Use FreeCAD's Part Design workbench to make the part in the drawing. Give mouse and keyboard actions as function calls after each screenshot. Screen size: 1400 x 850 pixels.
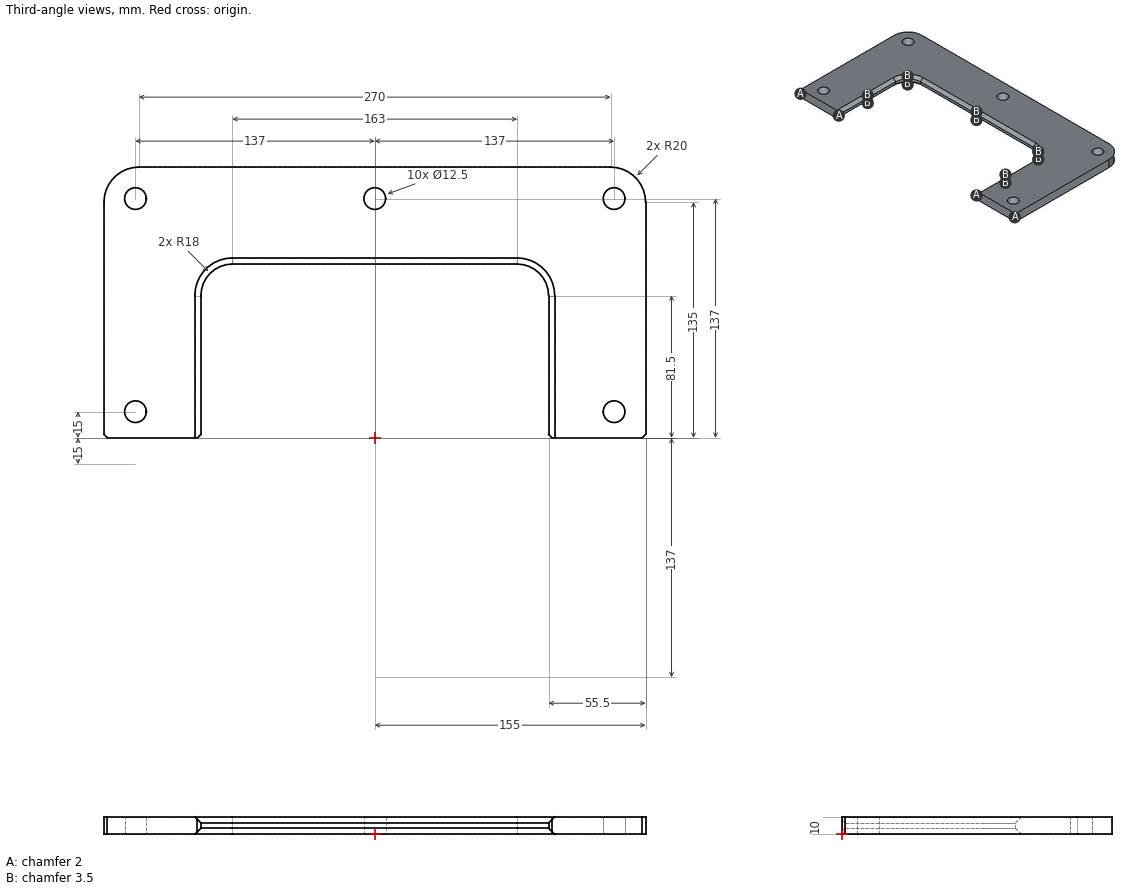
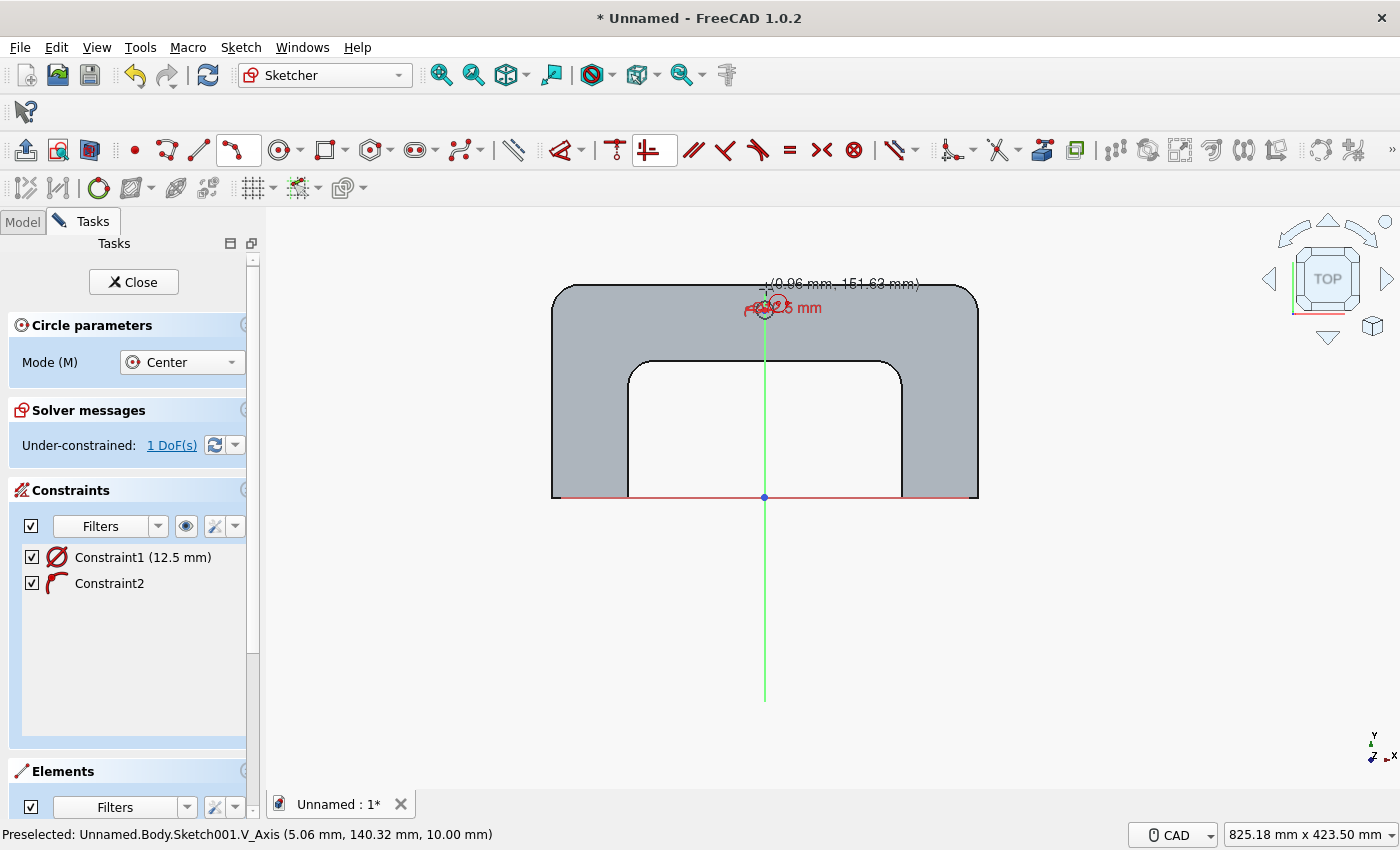
scroll(765, 686, up, 5)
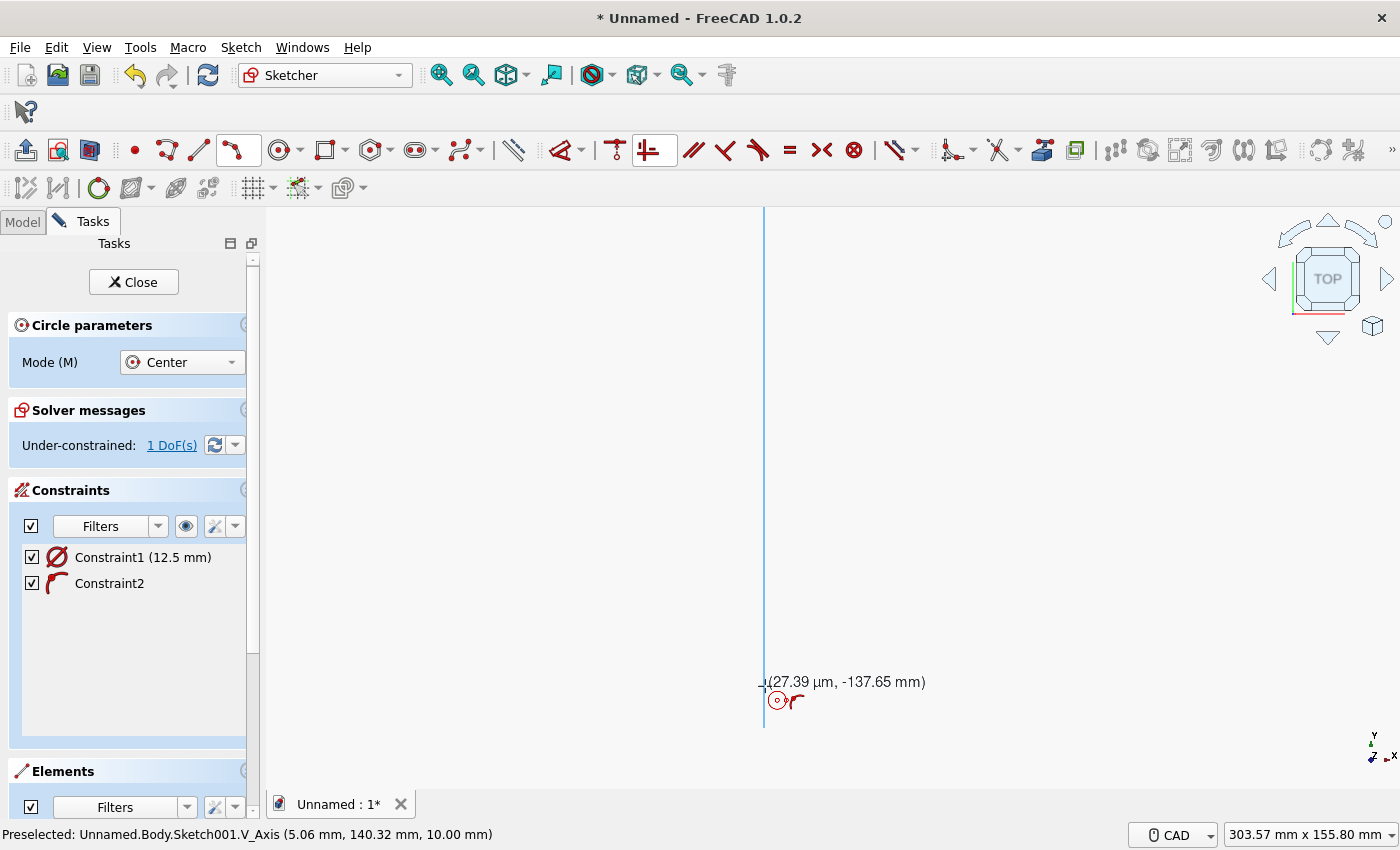
click(764, 685)
move(781, 668)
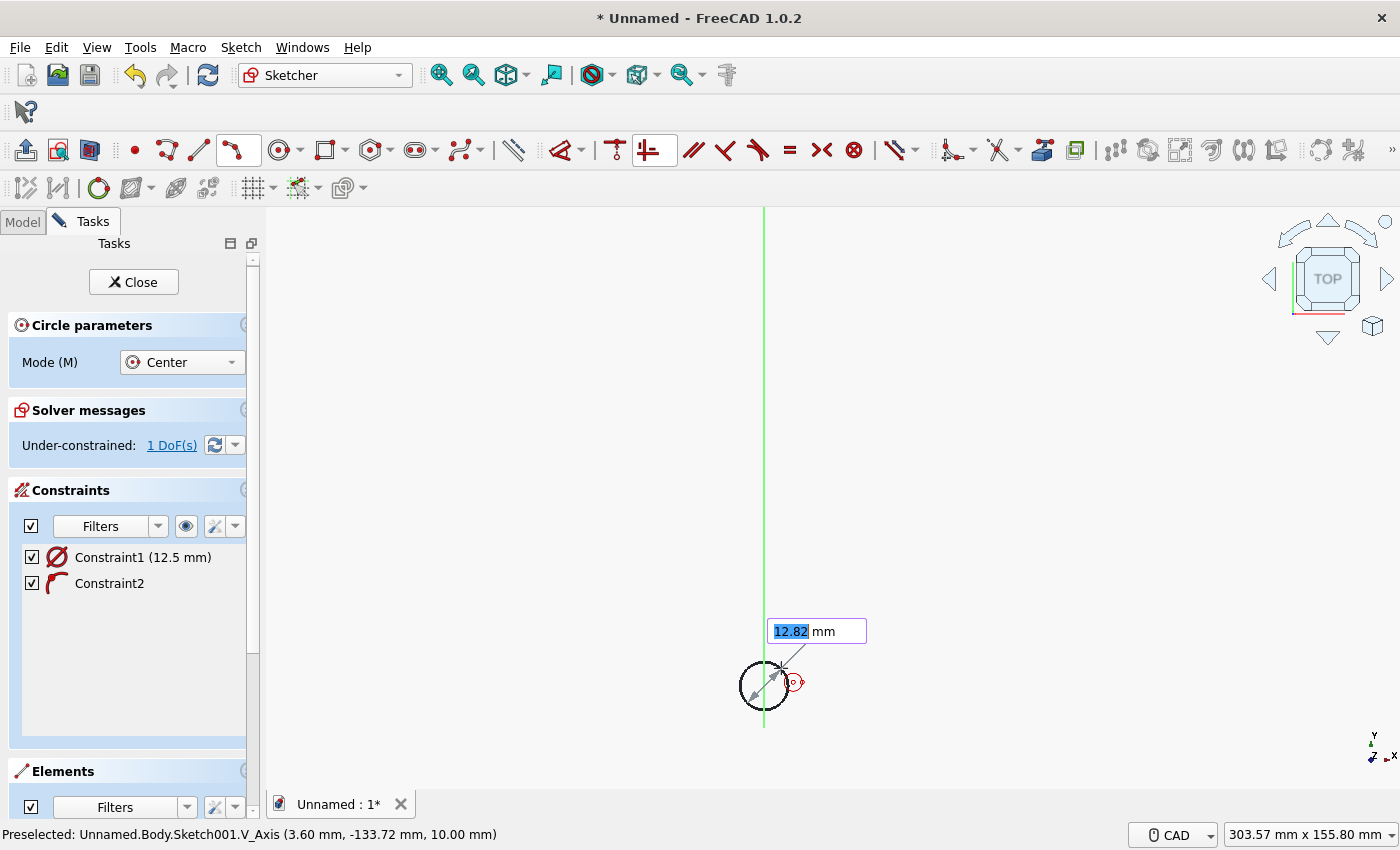
text(12.5)
key(Return)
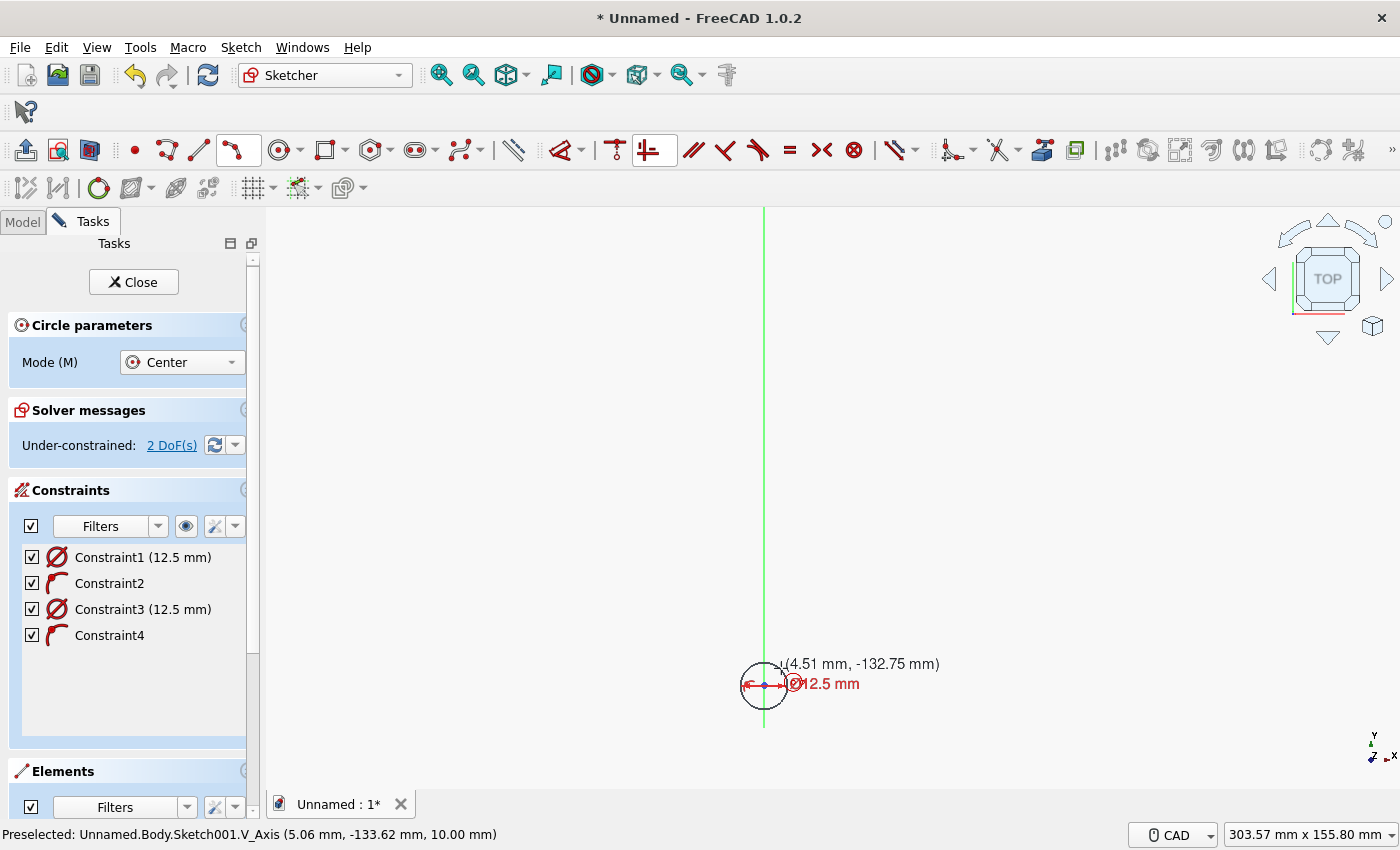
scroll(765, 687, down, 5)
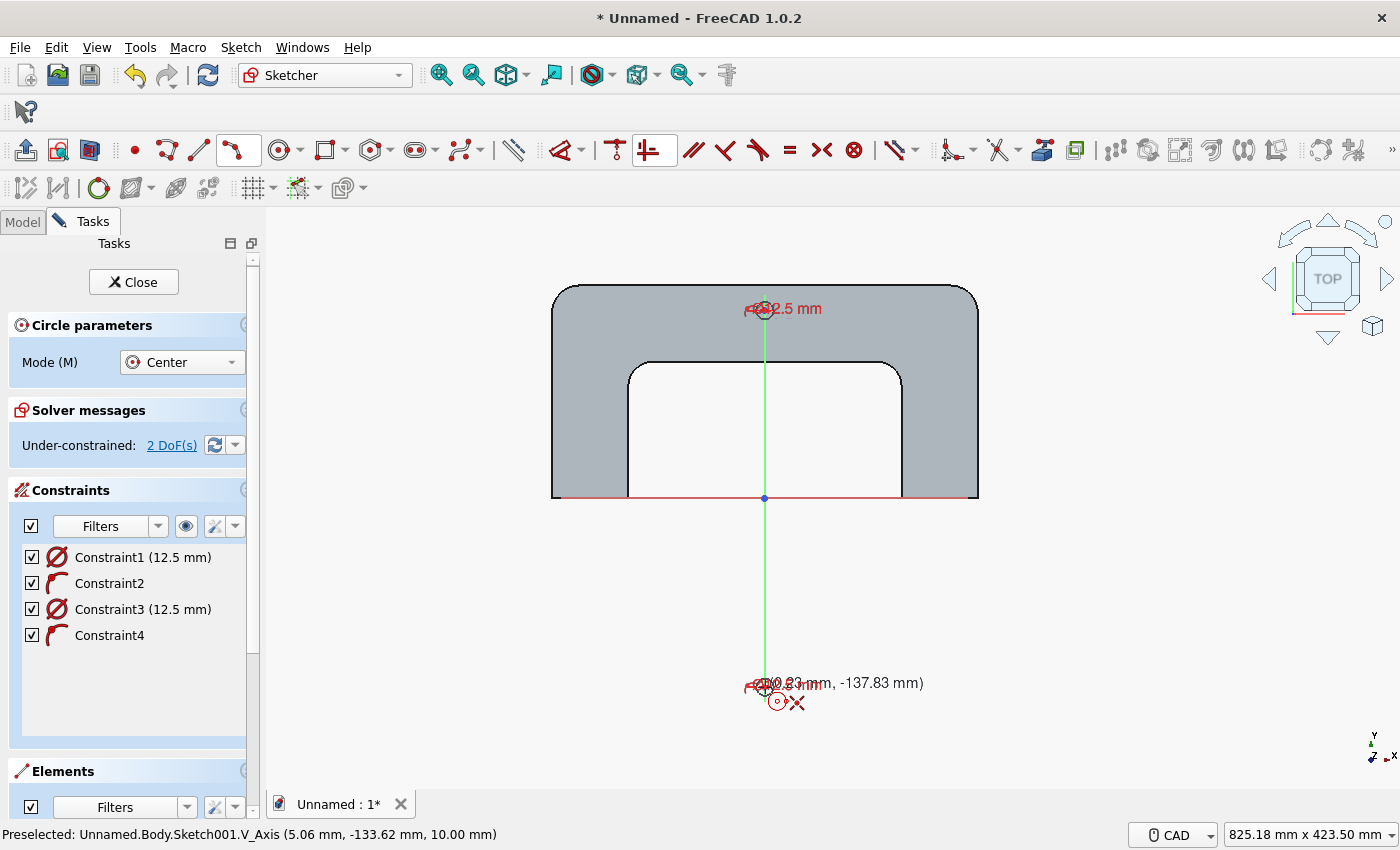
scroll(577, 310, up, 5)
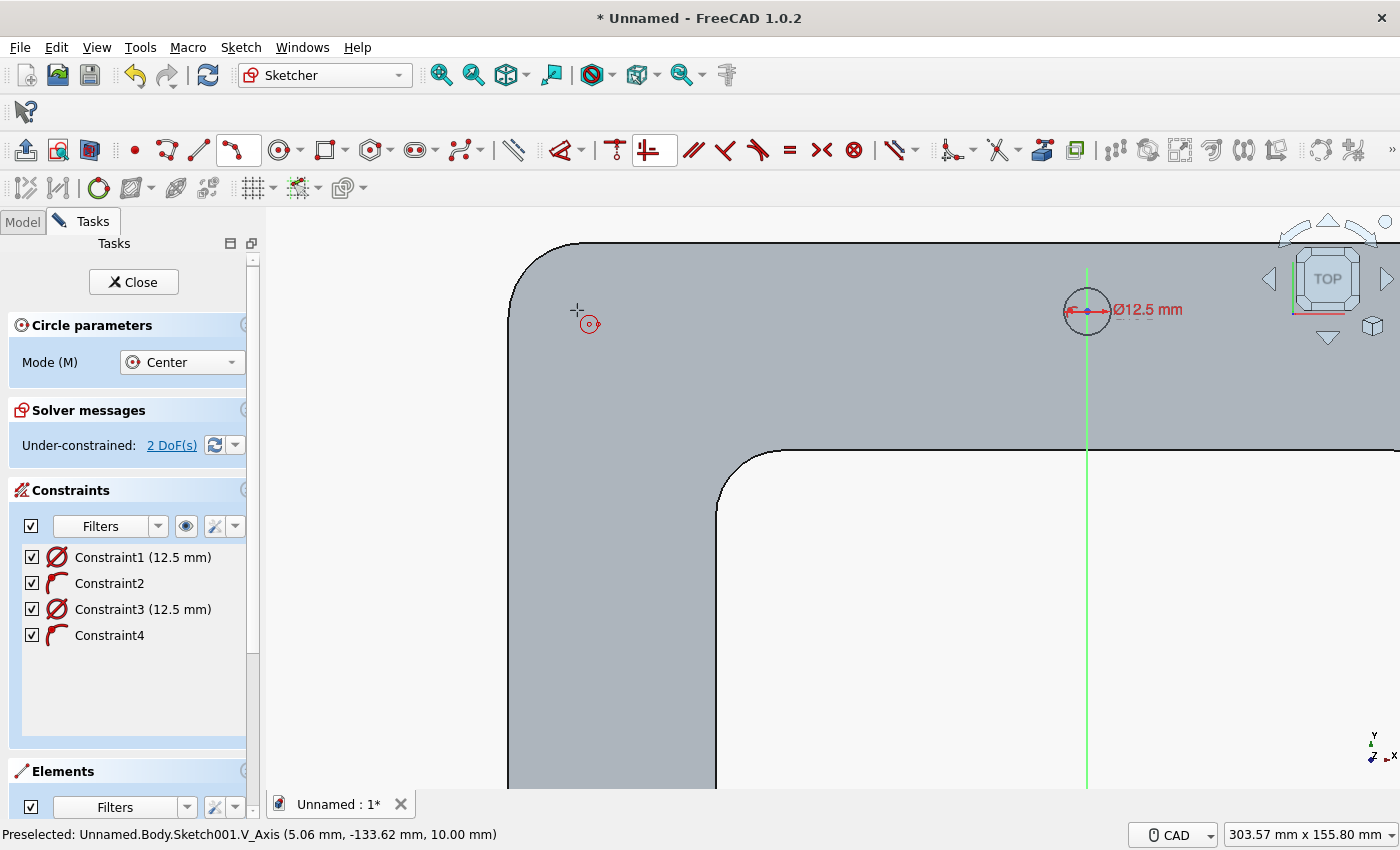
click(576, 310)
move(592, 294)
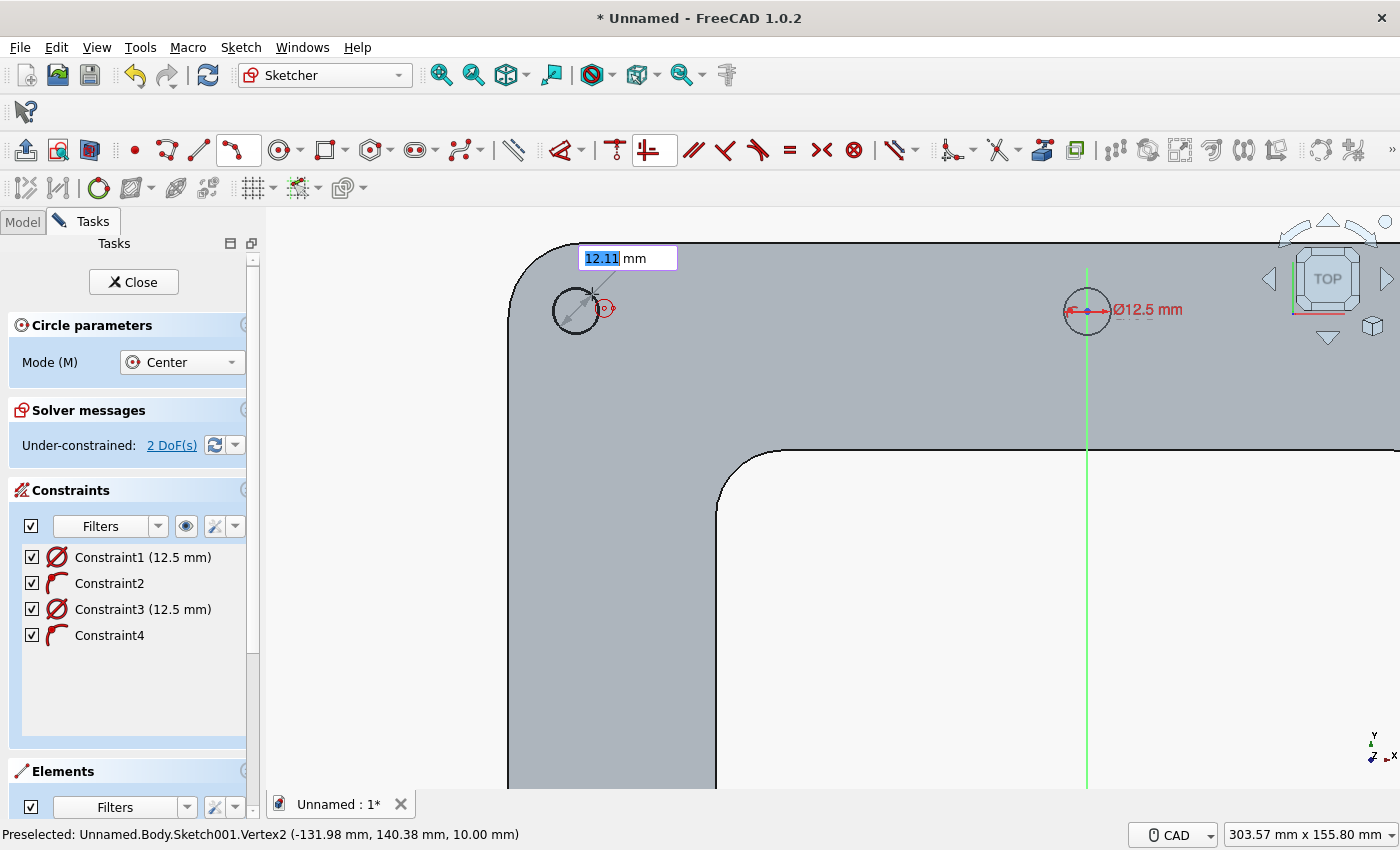
text(12.5)
key(Return)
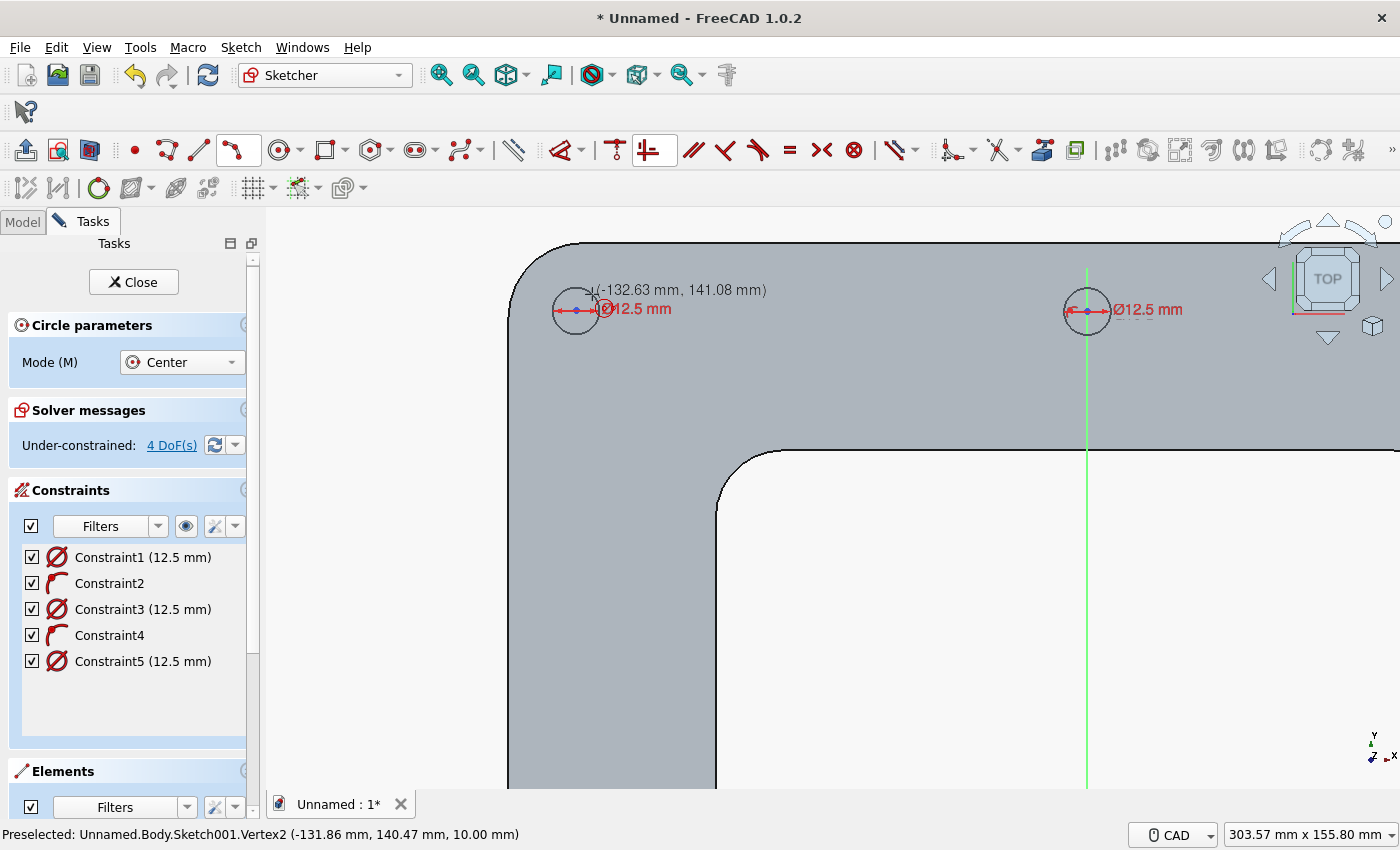
scroll(577, 309, down, 5)